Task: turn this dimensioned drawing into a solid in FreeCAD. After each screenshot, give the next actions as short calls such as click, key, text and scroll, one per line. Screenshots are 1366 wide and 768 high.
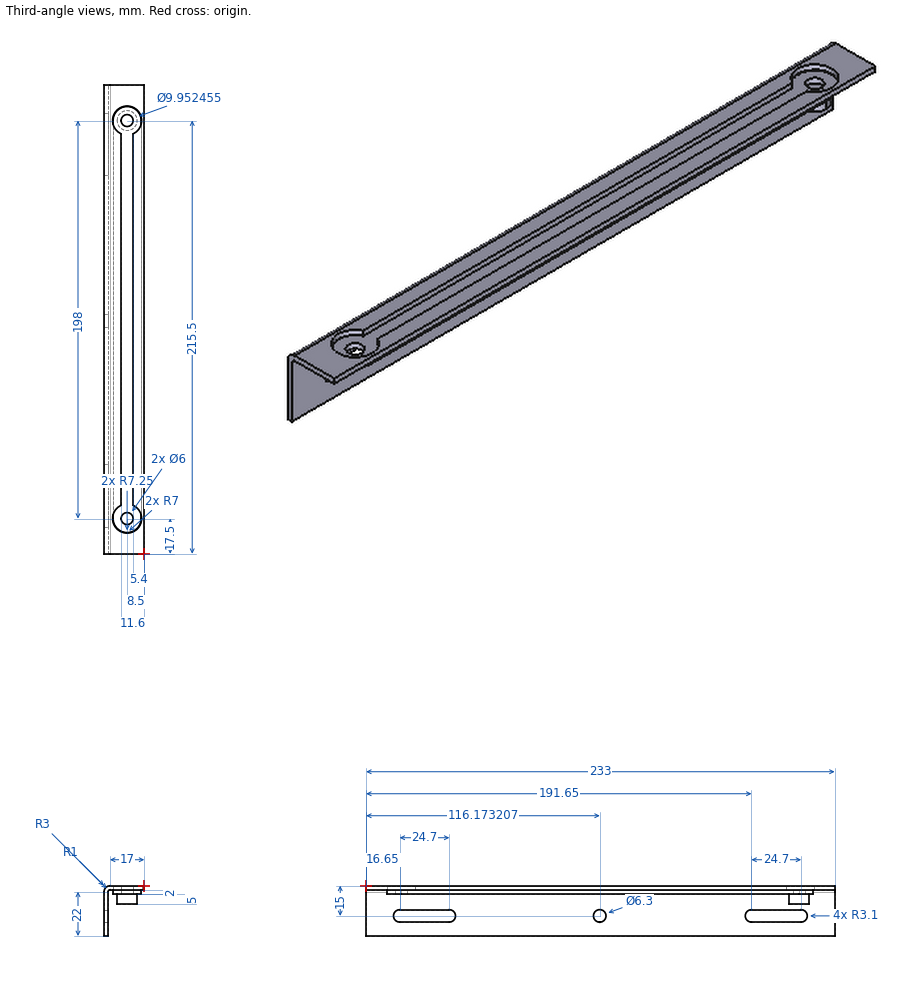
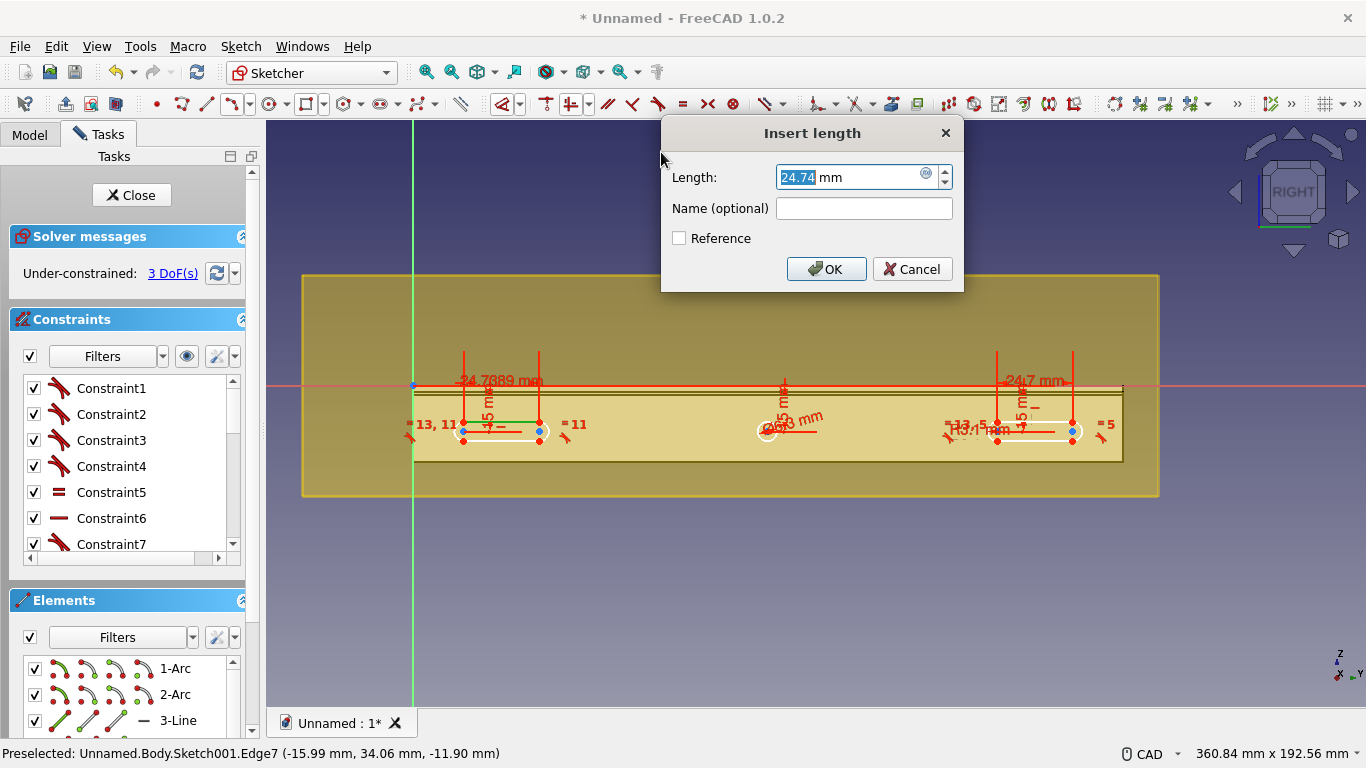
text(24.7)
key(Return)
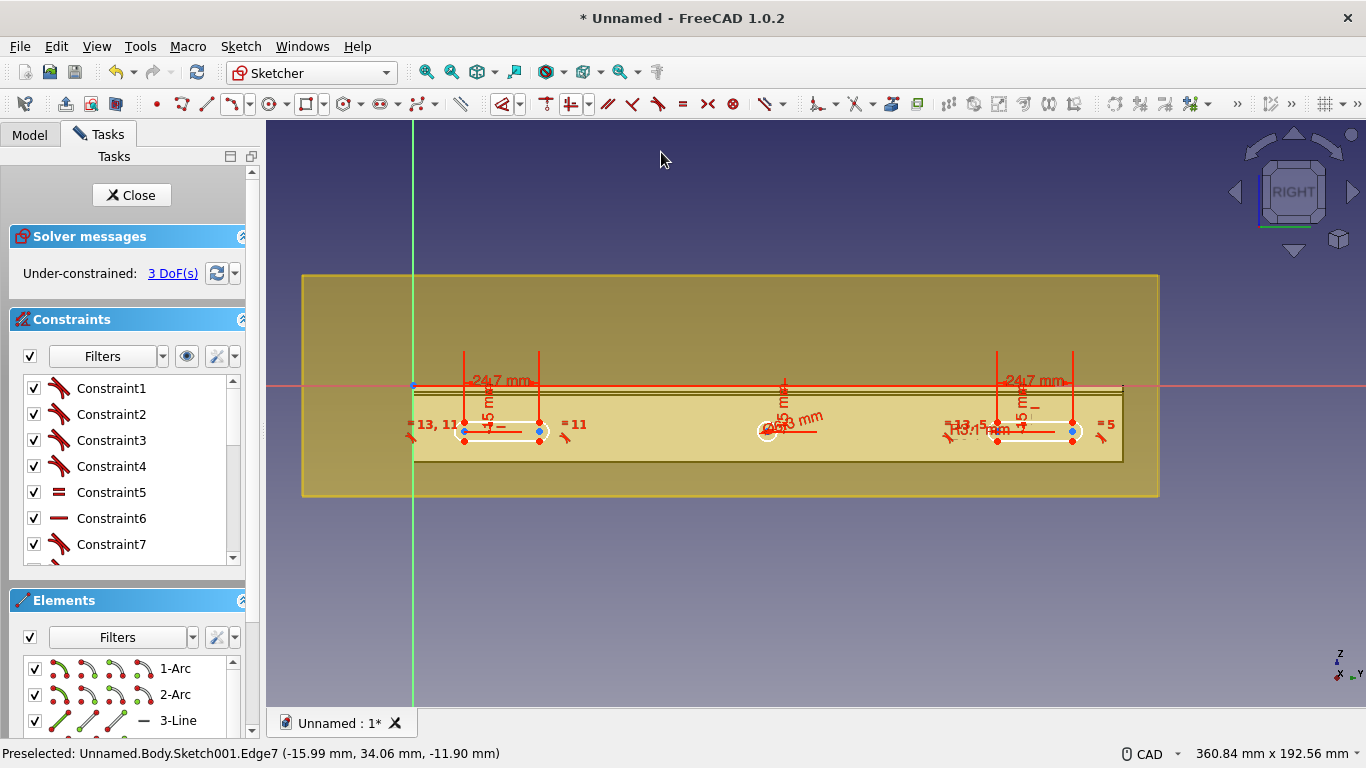
scroll(464, 422, up, 2)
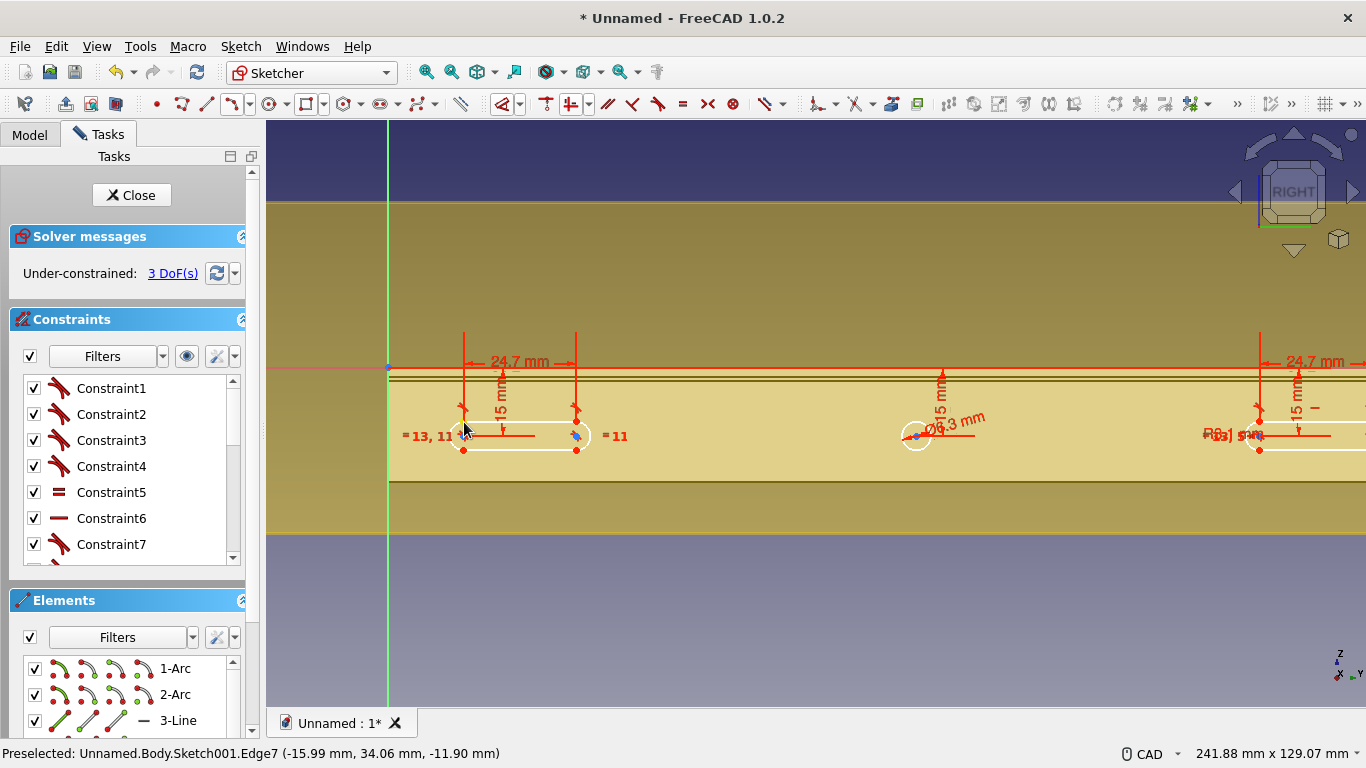
click(464, 422)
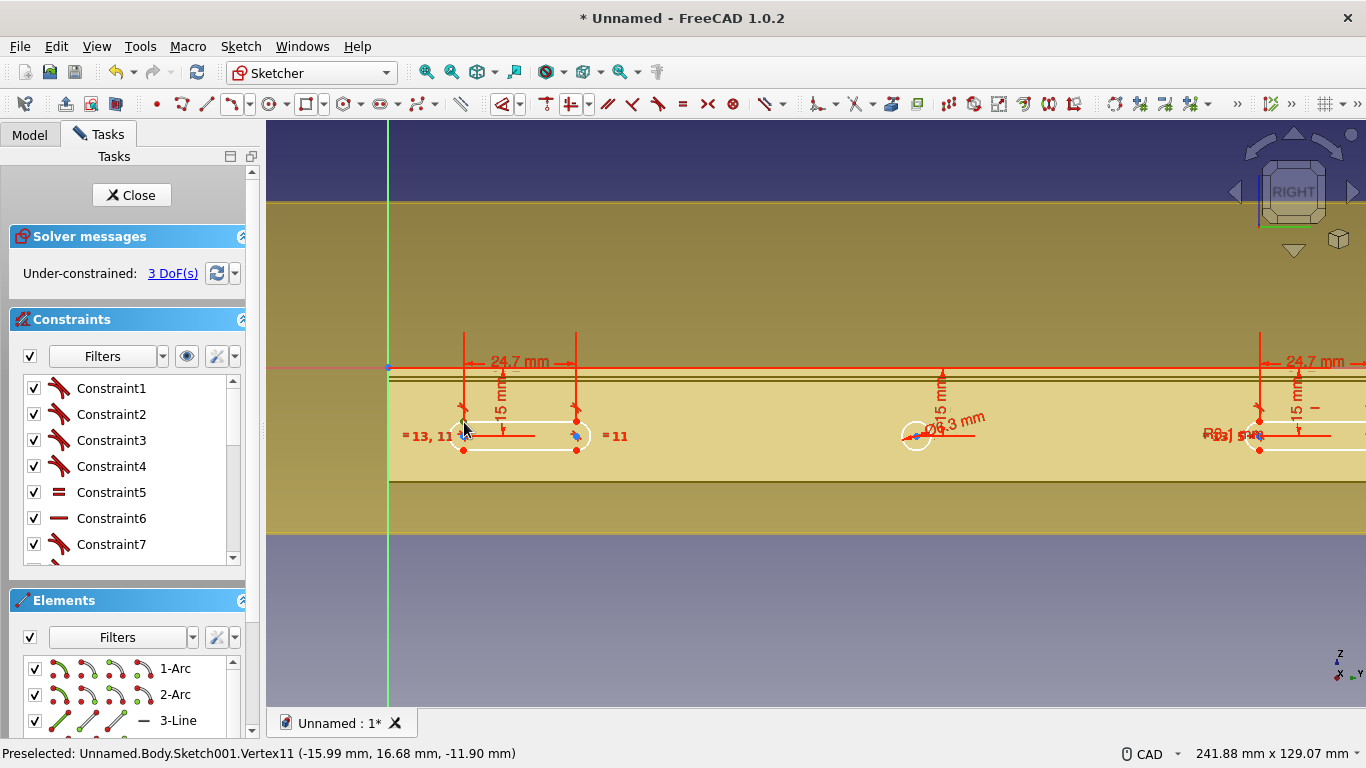
key(l)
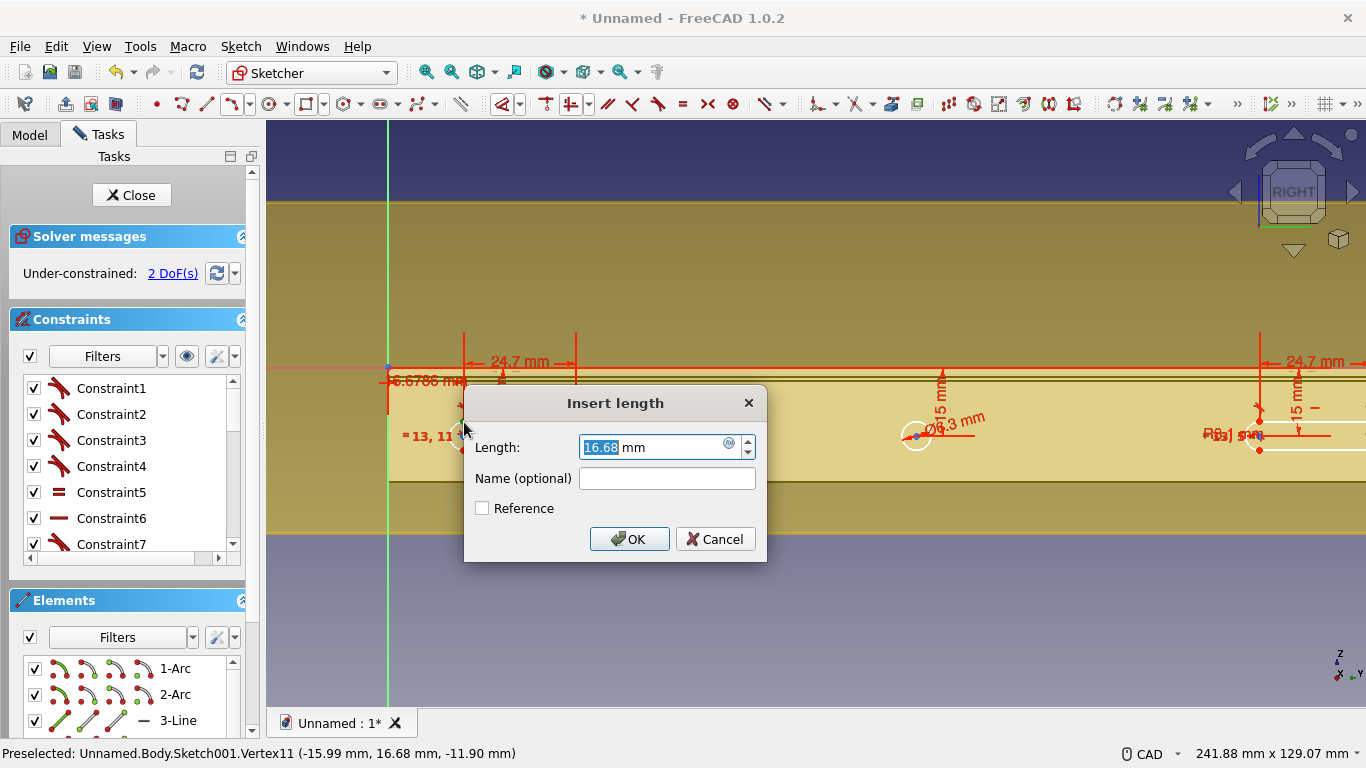
text(16.65)
key(Return)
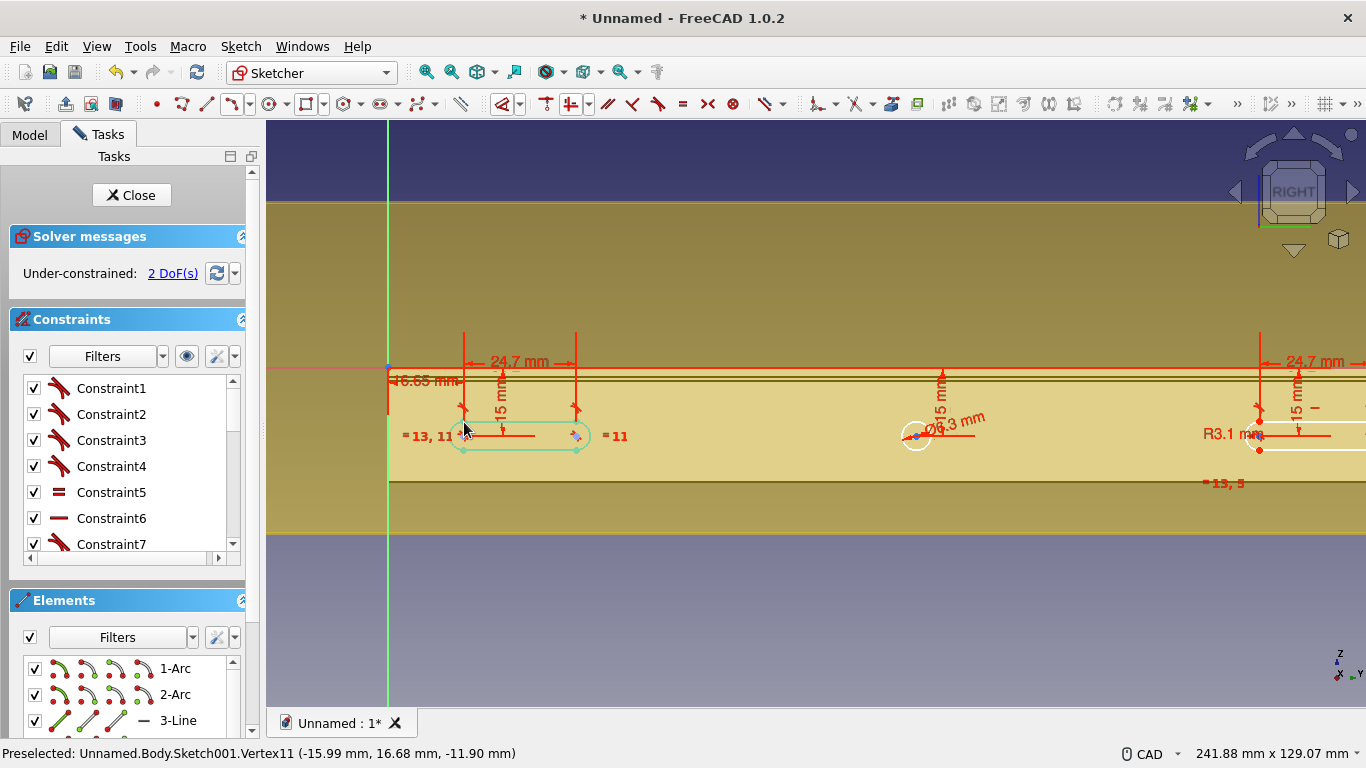
scroll(464, 422, down, 2)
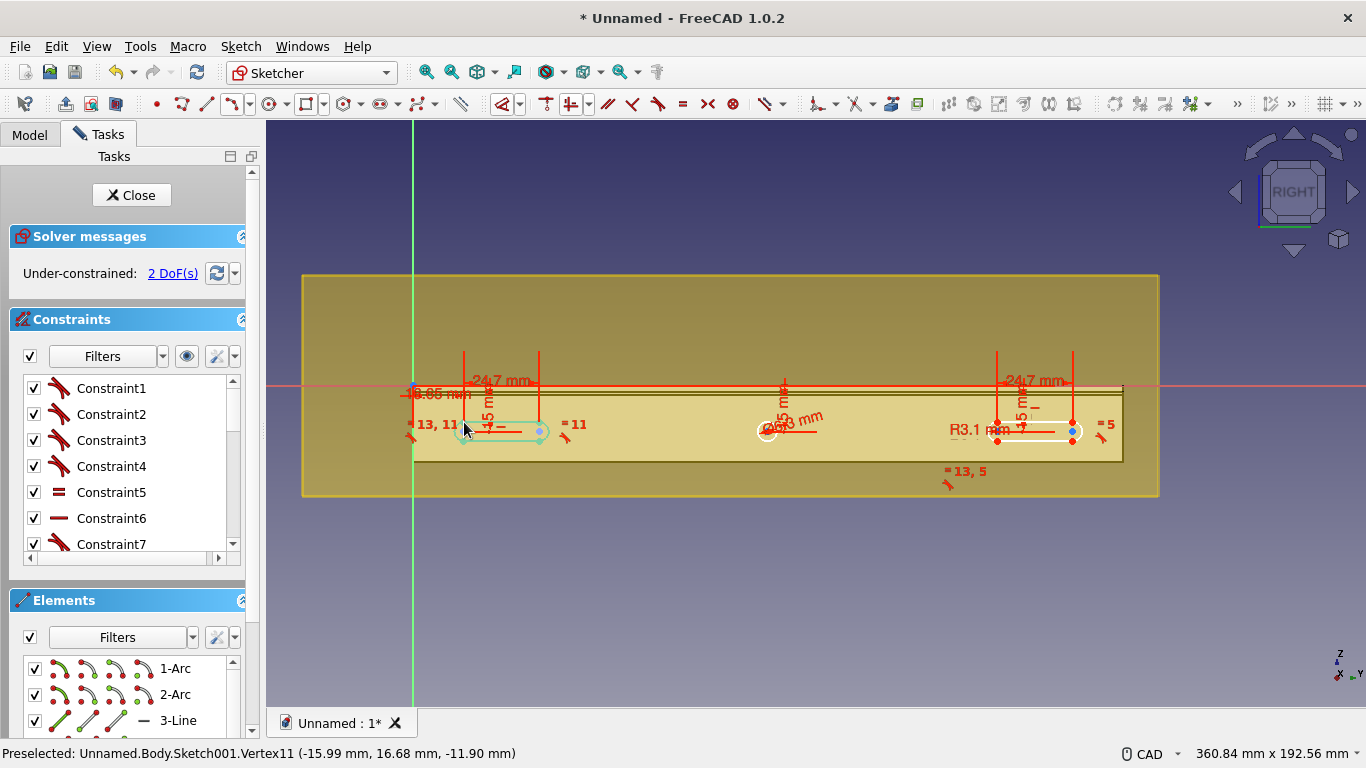
scroll(997, 422, up, 2)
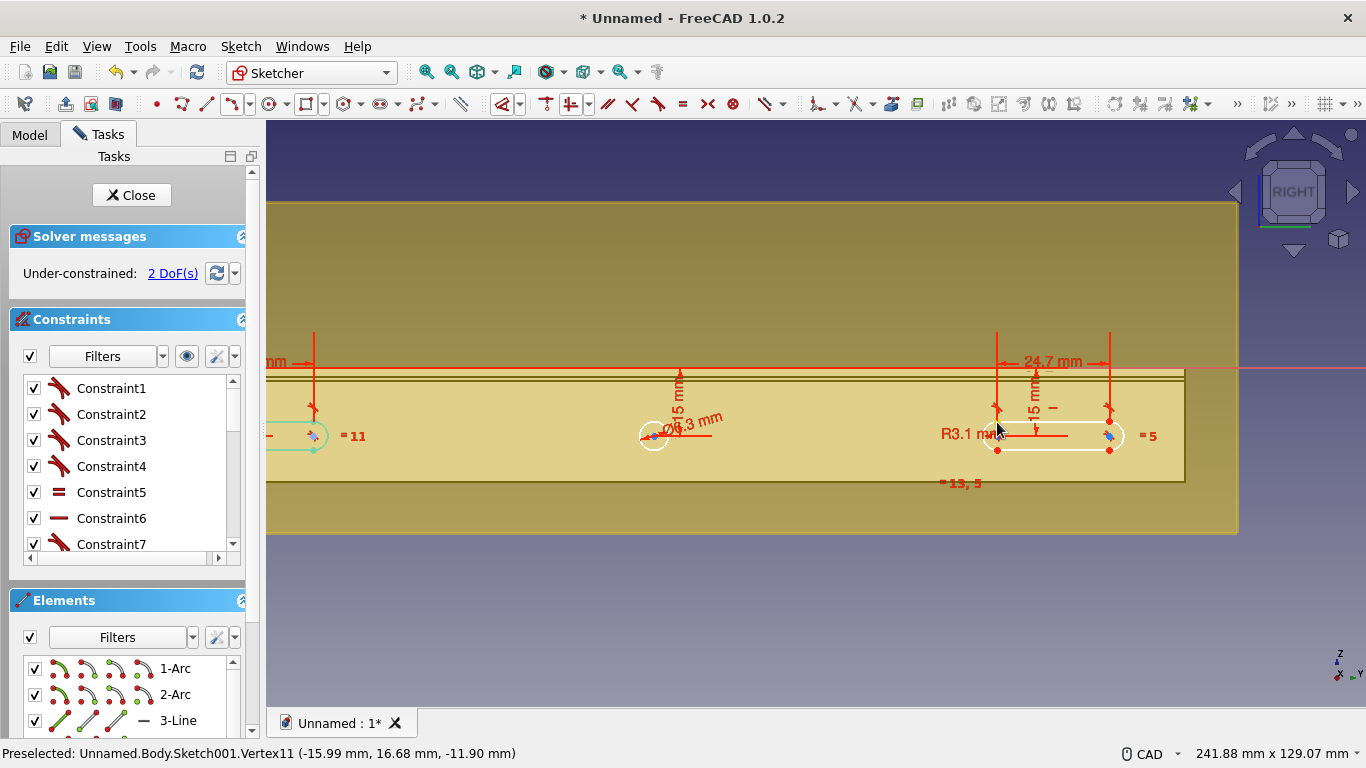
click(997, 422)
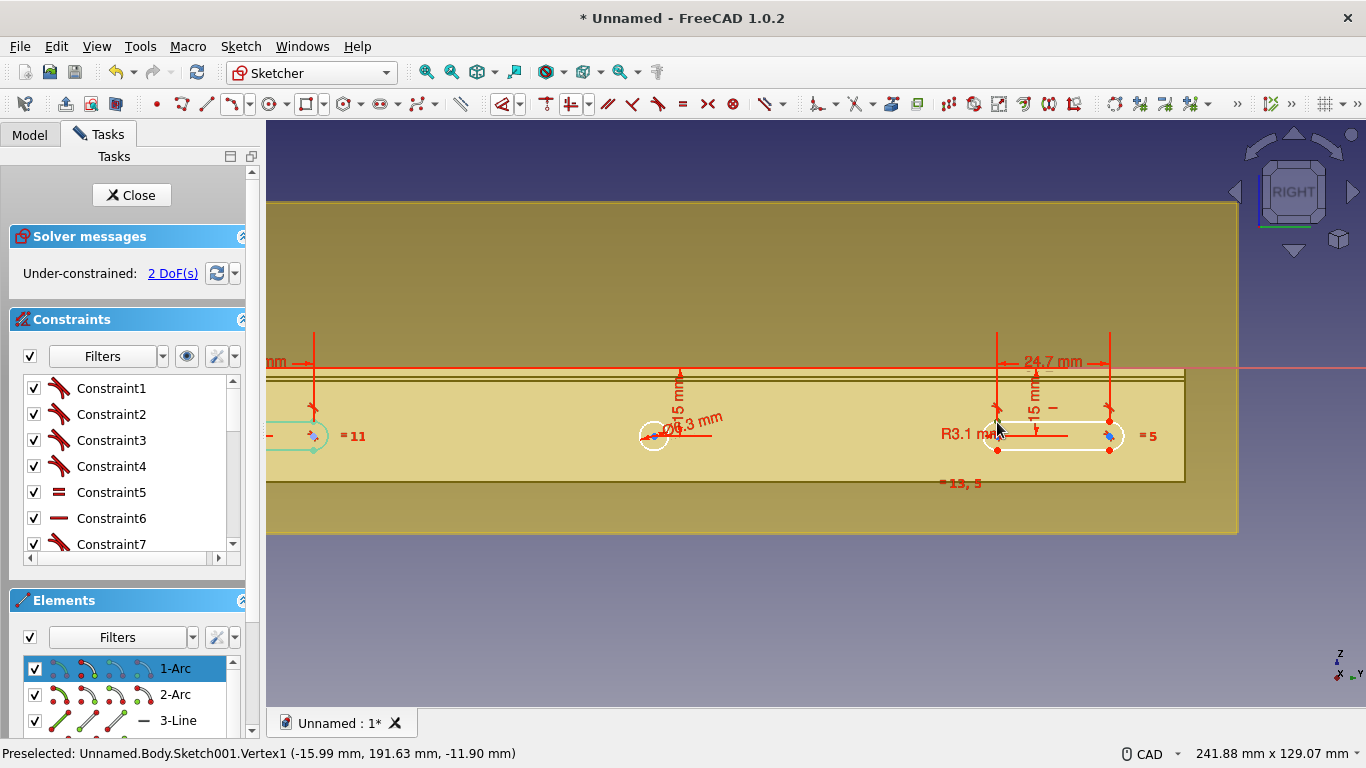
key(l)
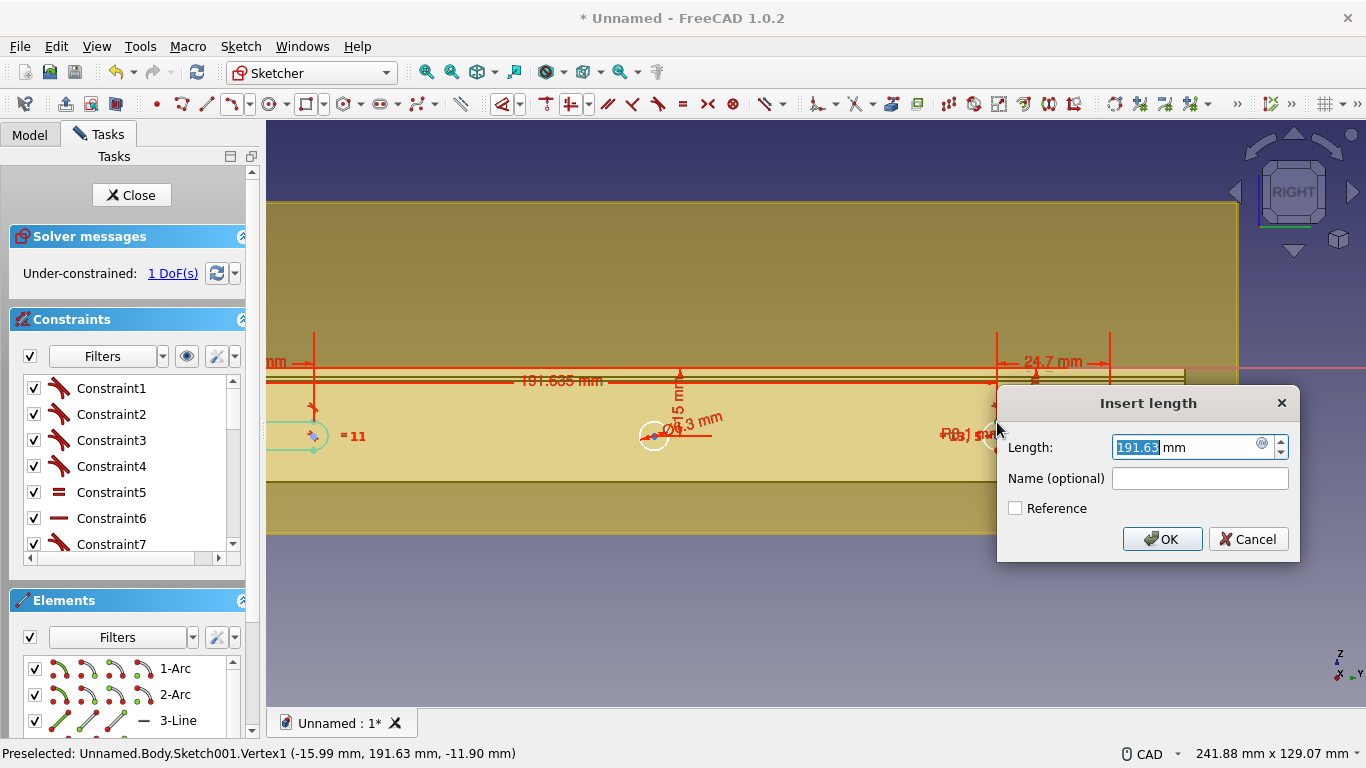
text(191.65)
key(Return)